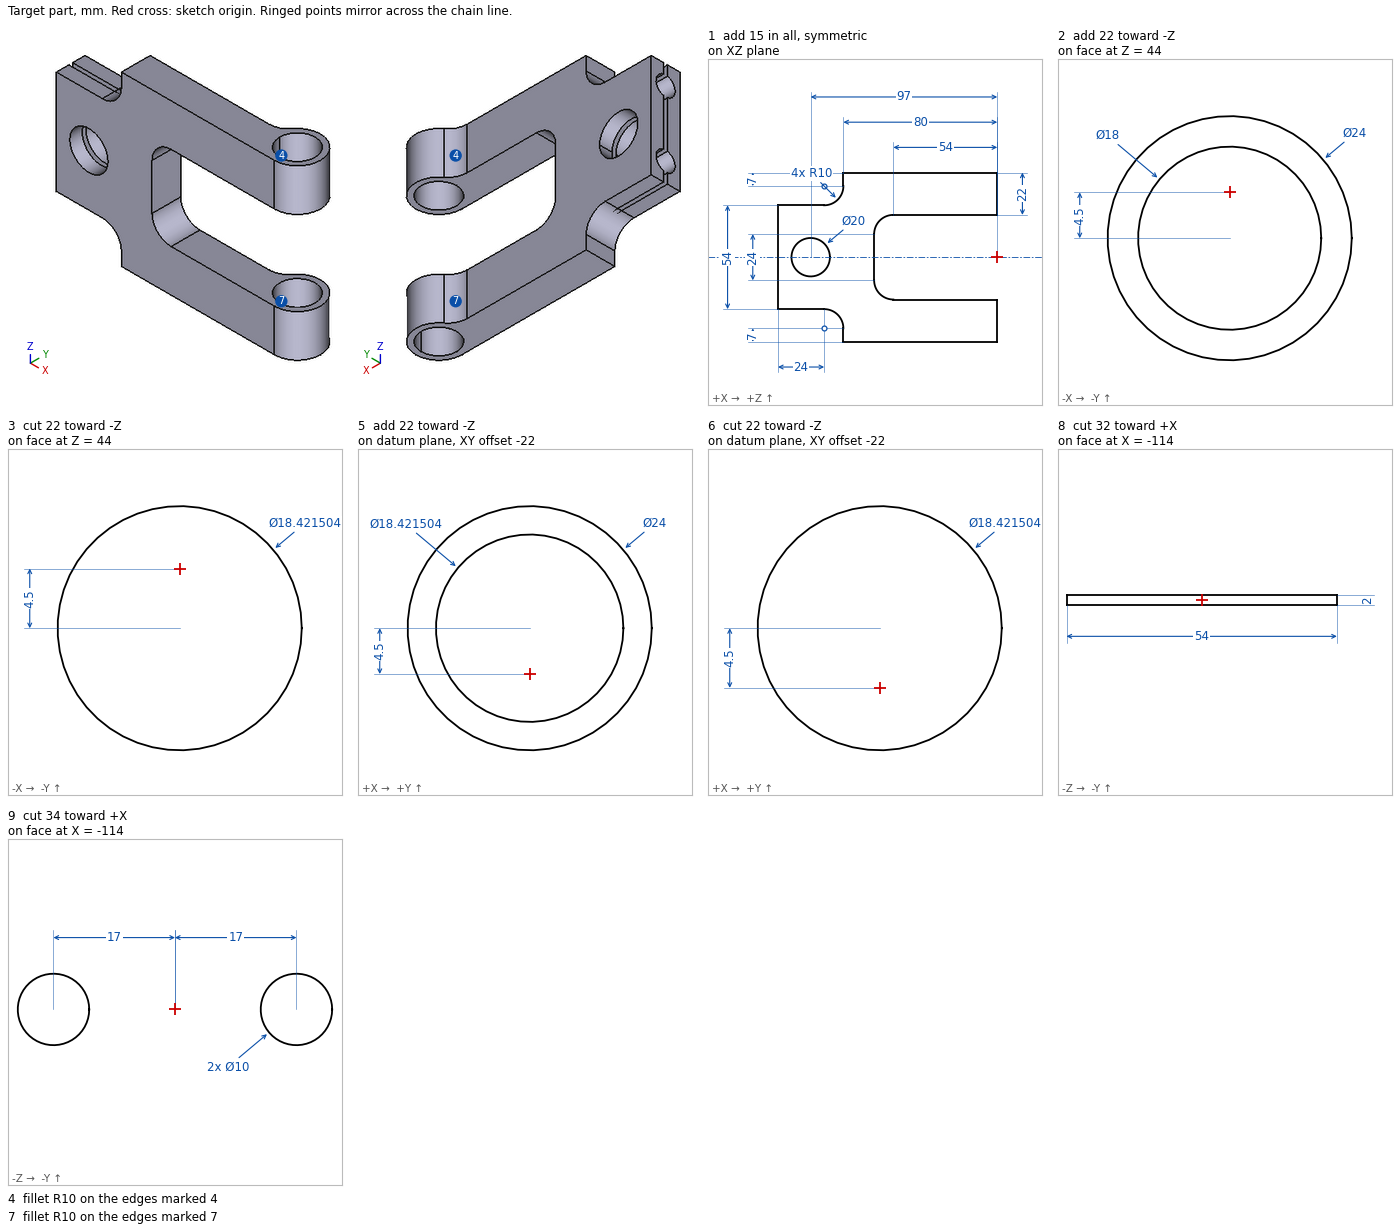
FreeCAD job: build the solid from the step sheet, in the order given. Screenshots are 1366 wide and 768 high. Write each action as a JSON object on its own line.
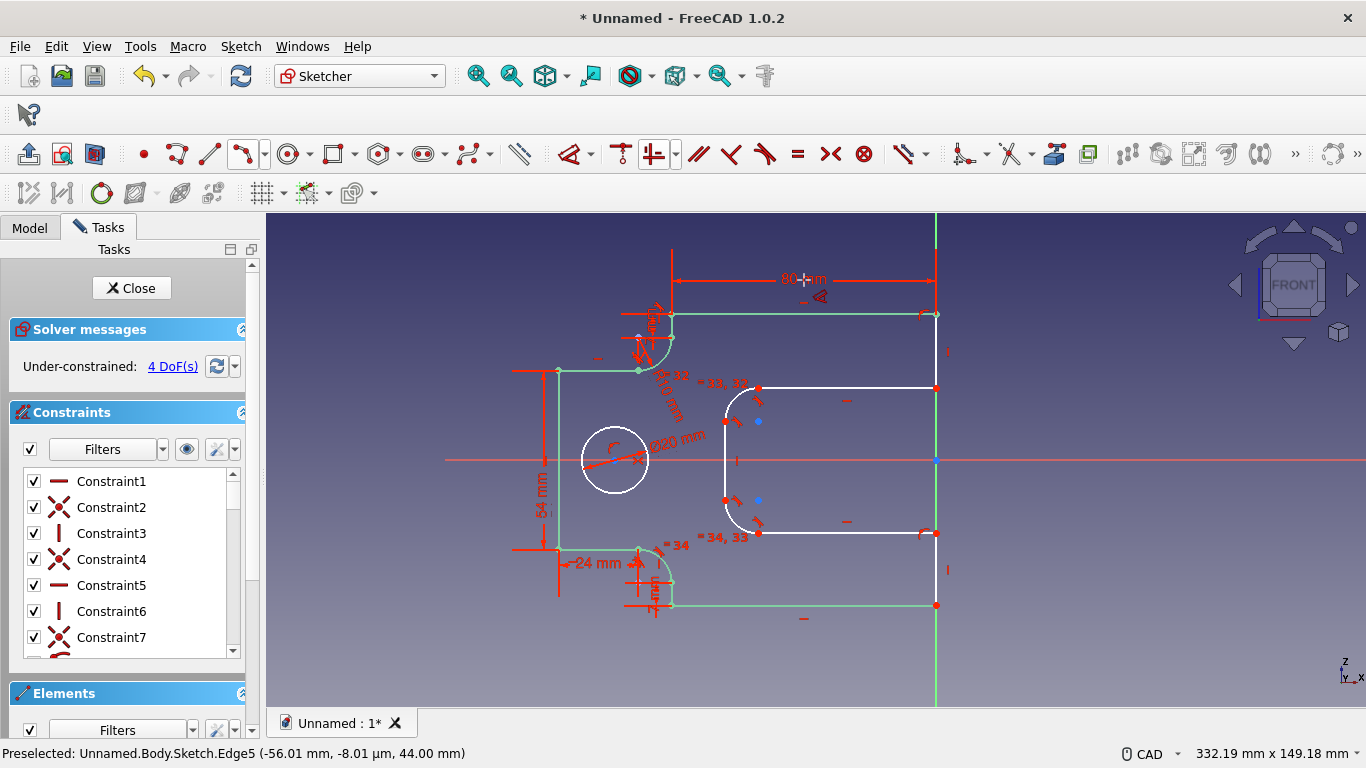
{"action": "left_click", "coordinate": [936, 337]}
{"action": "left_click", "coordinate": [970, 351]}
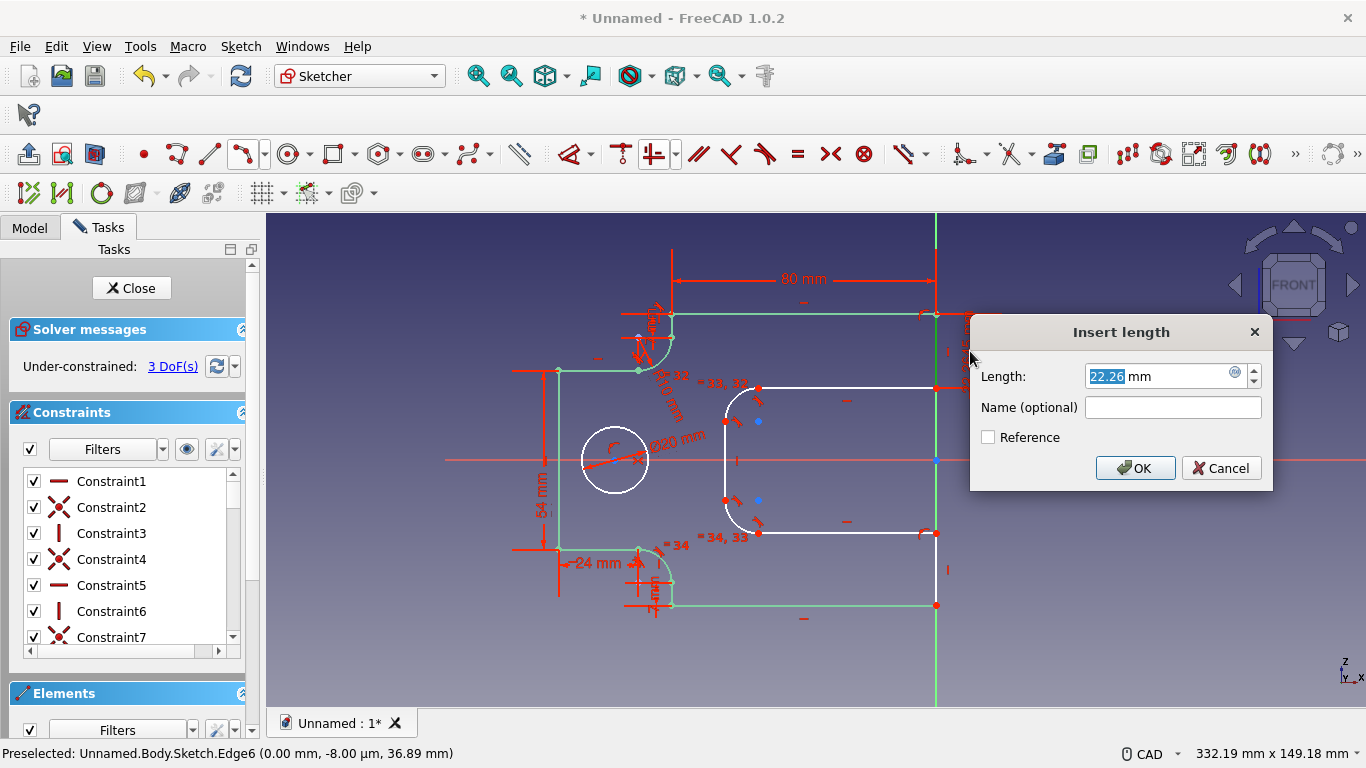
{"action": "type", "text": "22"}
{"action": "key", "text": "Return"}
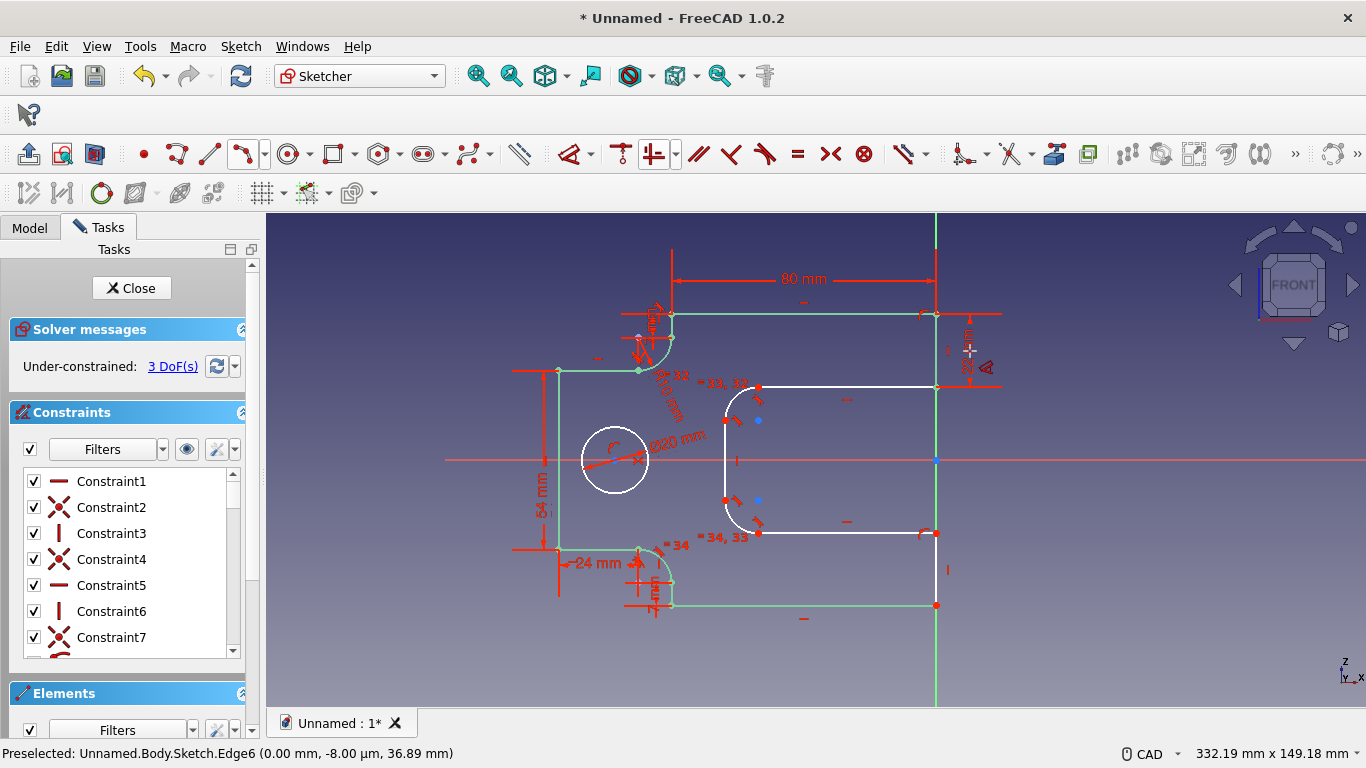
{"action": "left_click", "coordinate": [883, 387]}
{"action": "left_click", "coordinate": [848, 353]}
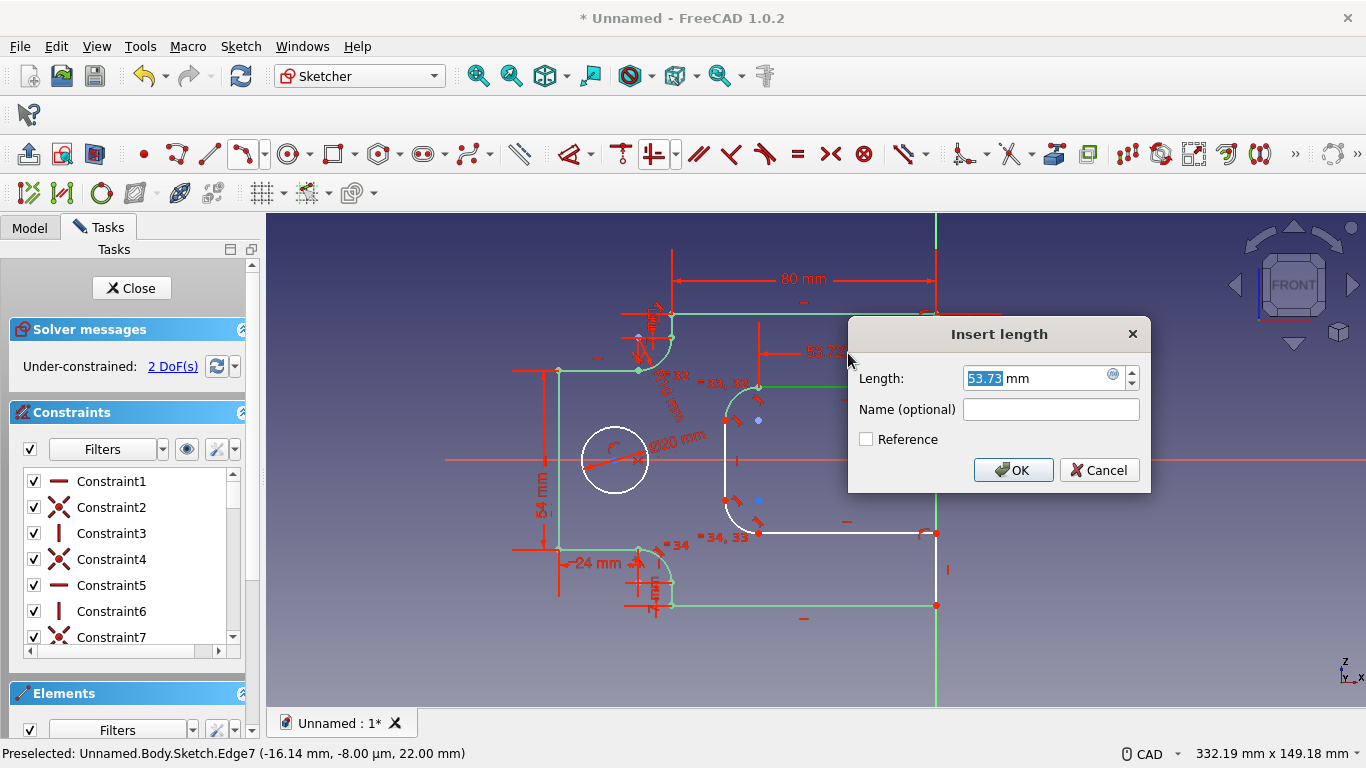
{"action": "type", "text": "54"}
{"action": "key", "text": "Return"}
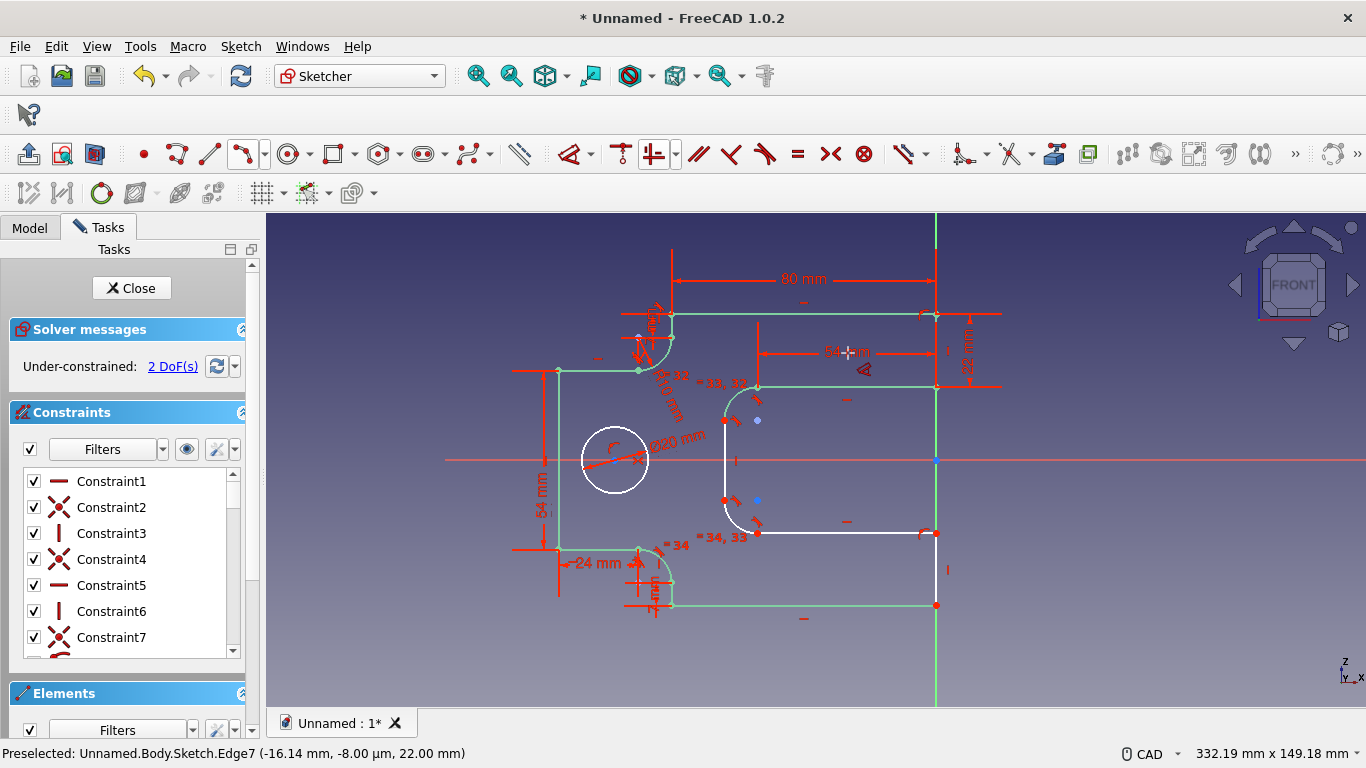
{"action": "left_click", "coordinate": [725, 444]}
{"action": "left_click", "coordinate": [691, 479]}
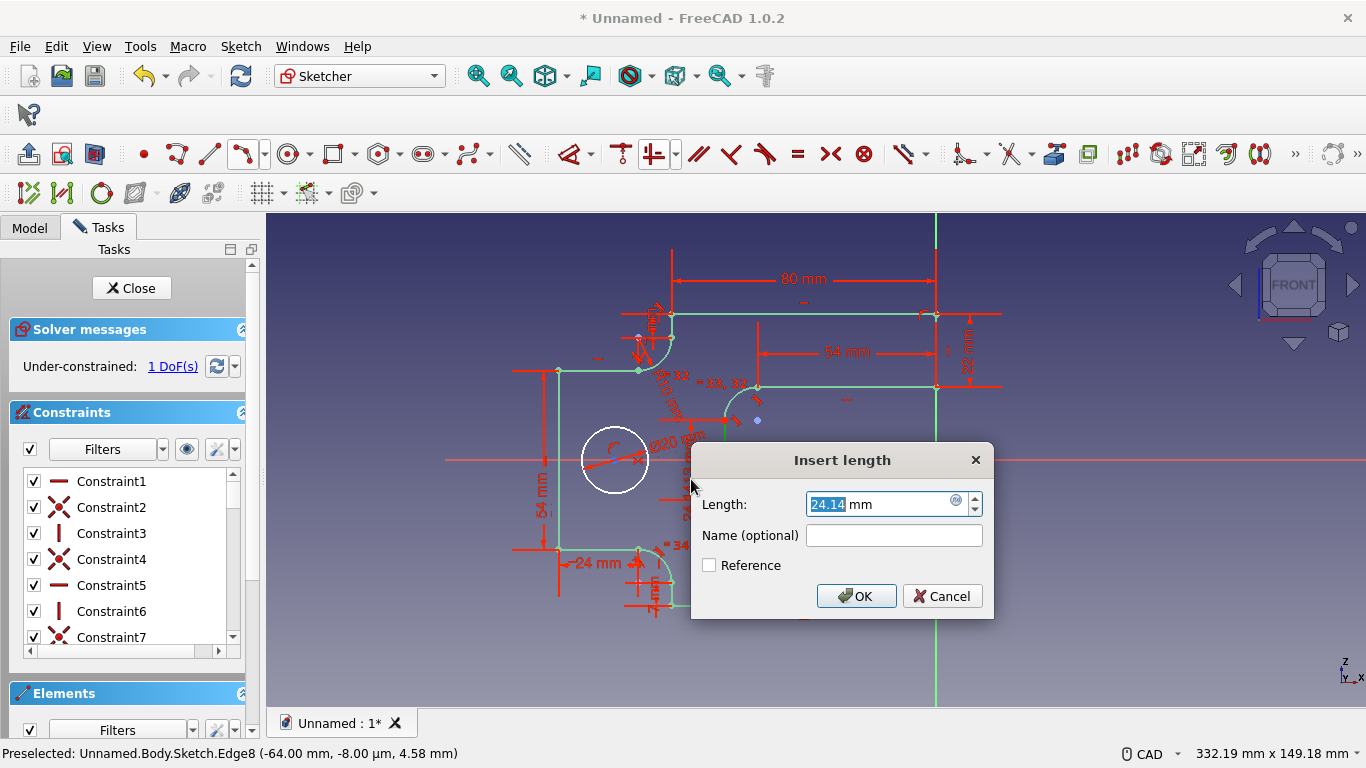
{"action": "type", "text": "24"}
{"action": "key", "text": "Return"}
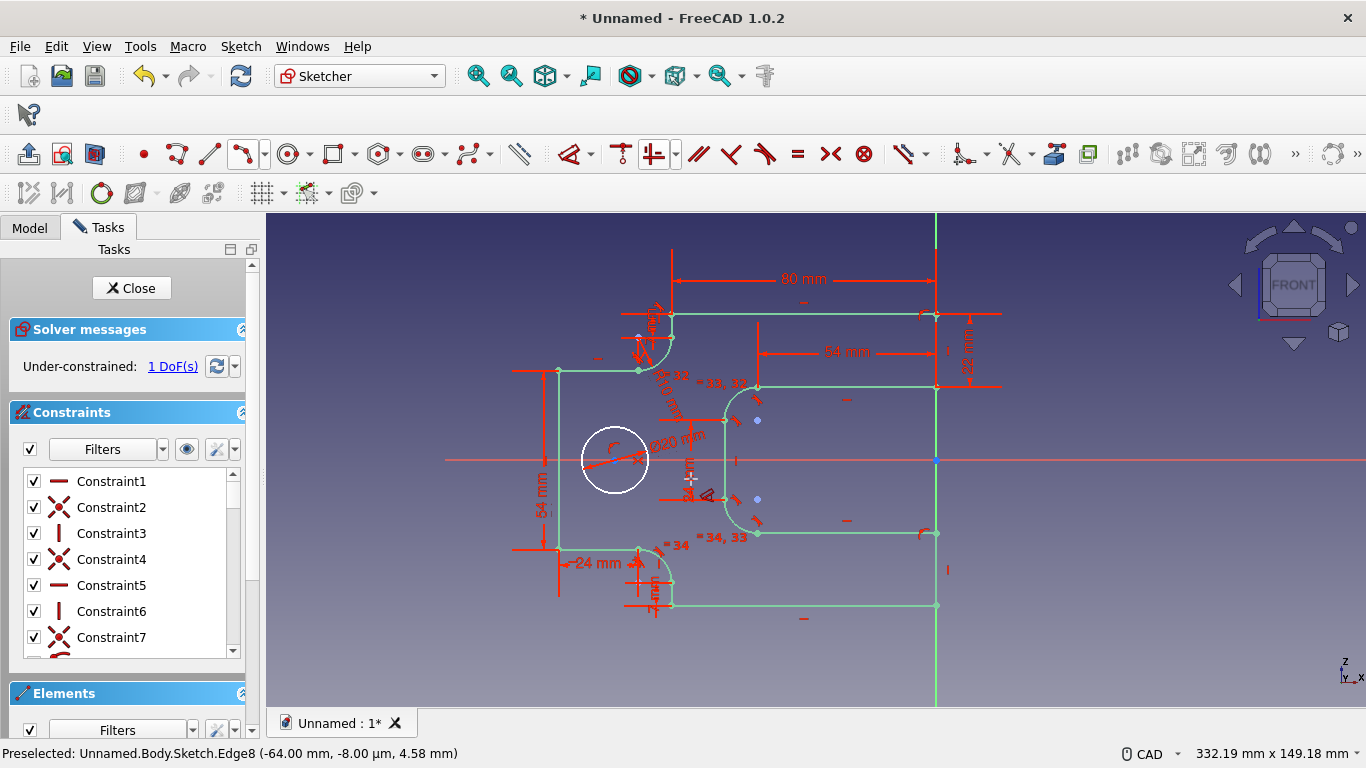
{"action": "left_click", "coordinate": [615, 460]}
{"action": "left_click", "coordinate": [776, 494]}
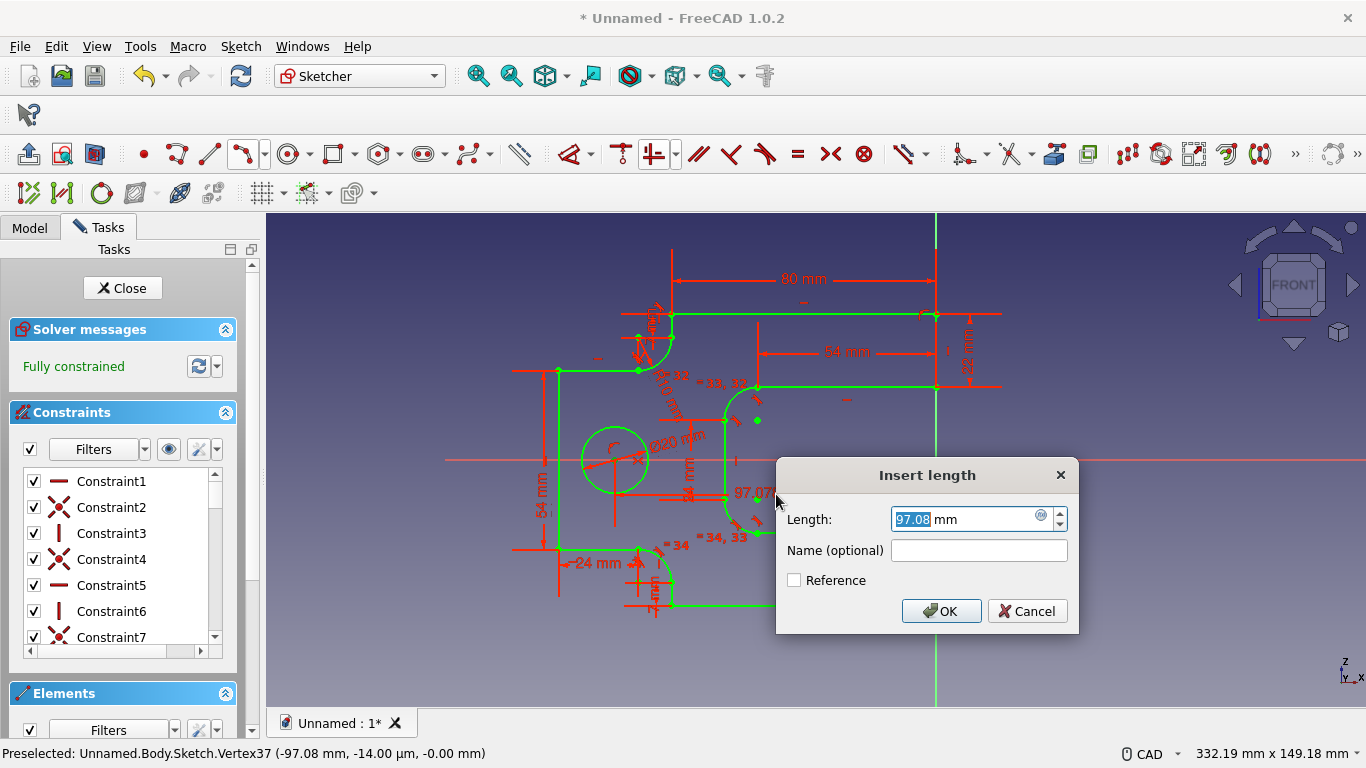
{"action": "type", "text": "97"}
{"action": "key", "text": "Return"}
{"action": "key", "text": "Escape"}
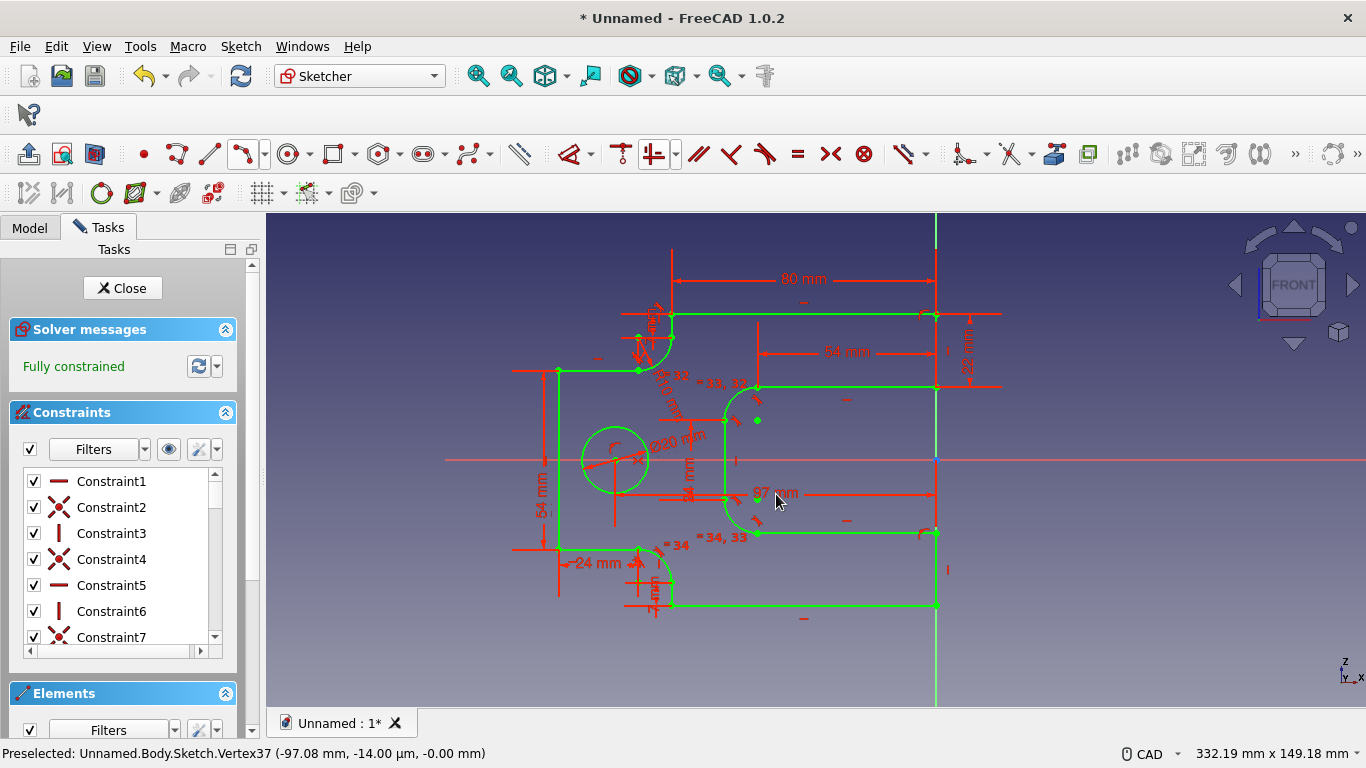
{"action": "left_click", "coordinate": [123, 288]}